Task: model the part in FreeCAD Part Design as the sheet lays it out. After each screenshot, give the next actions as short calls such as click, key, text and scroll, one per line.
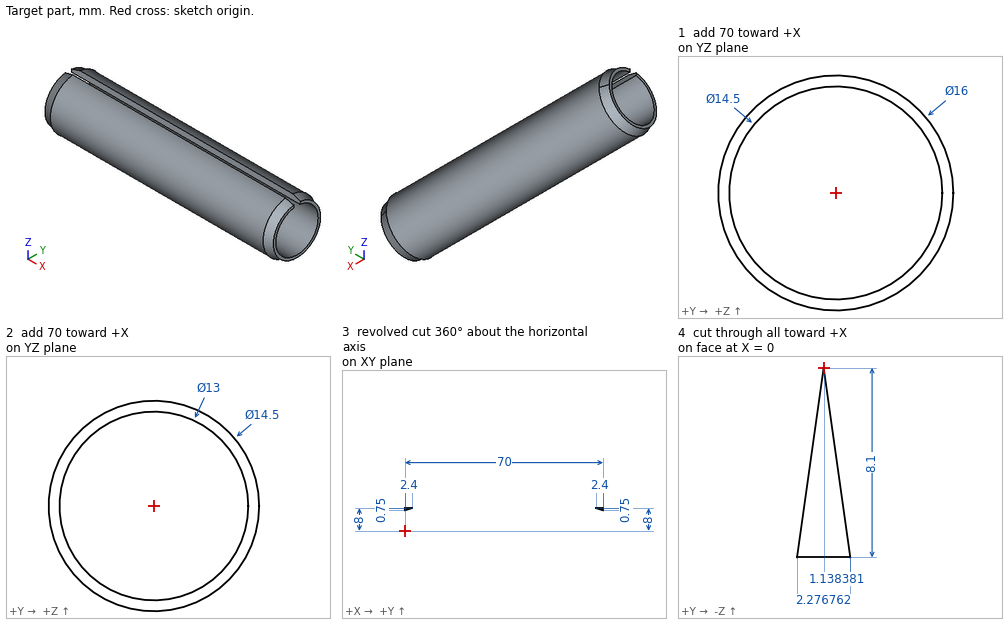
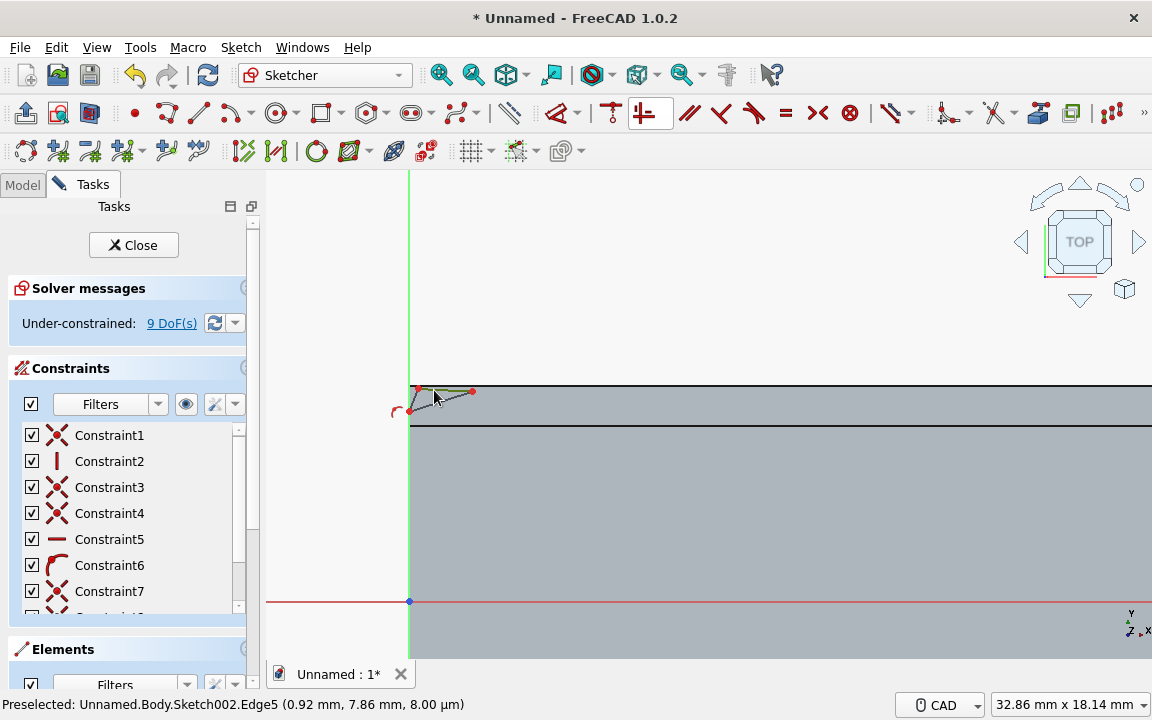
key(h)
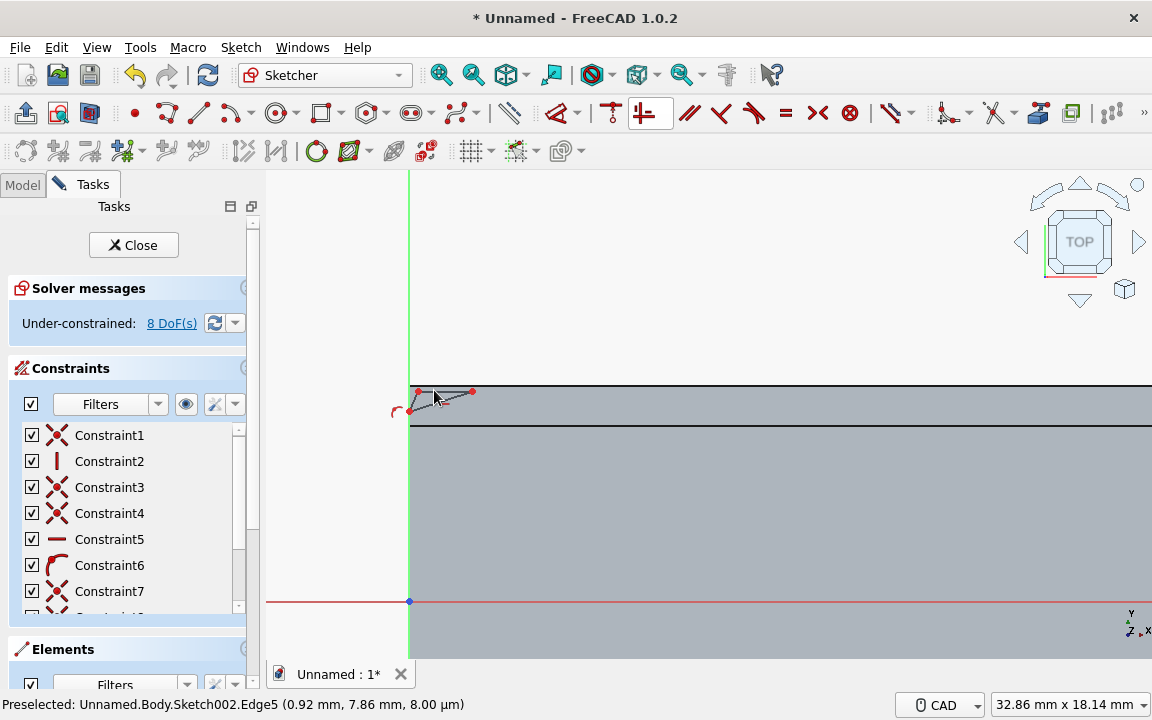
scroll(413, 404, up, 4)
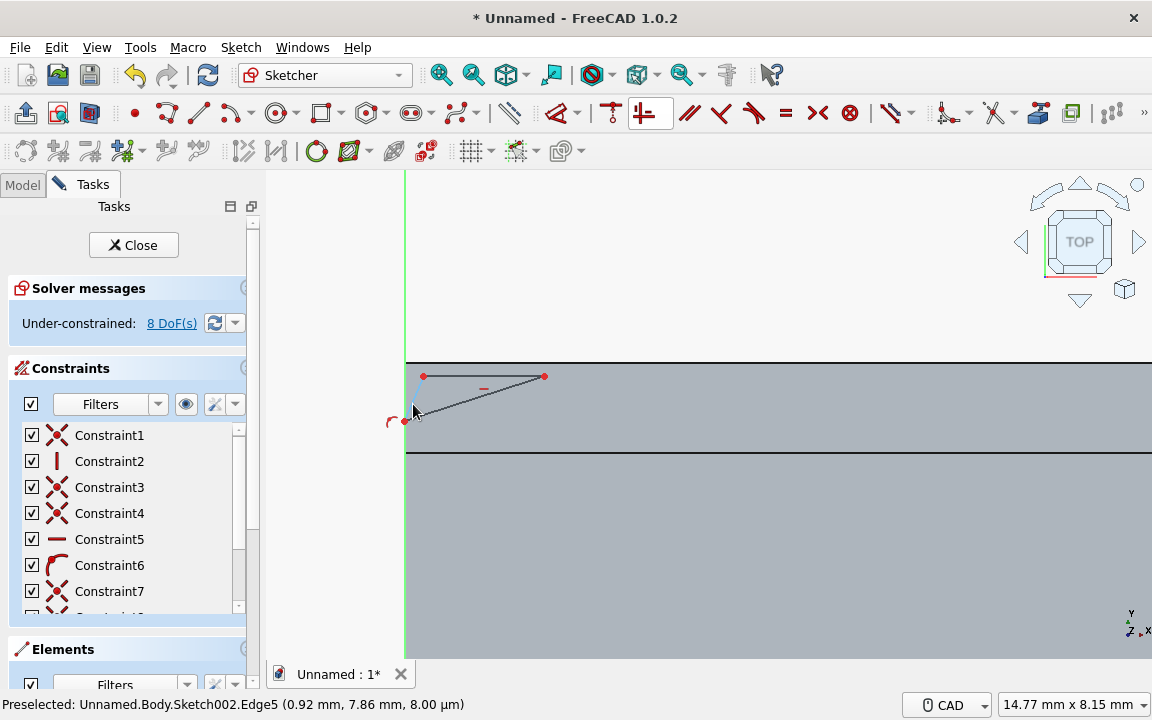
click(412, 403)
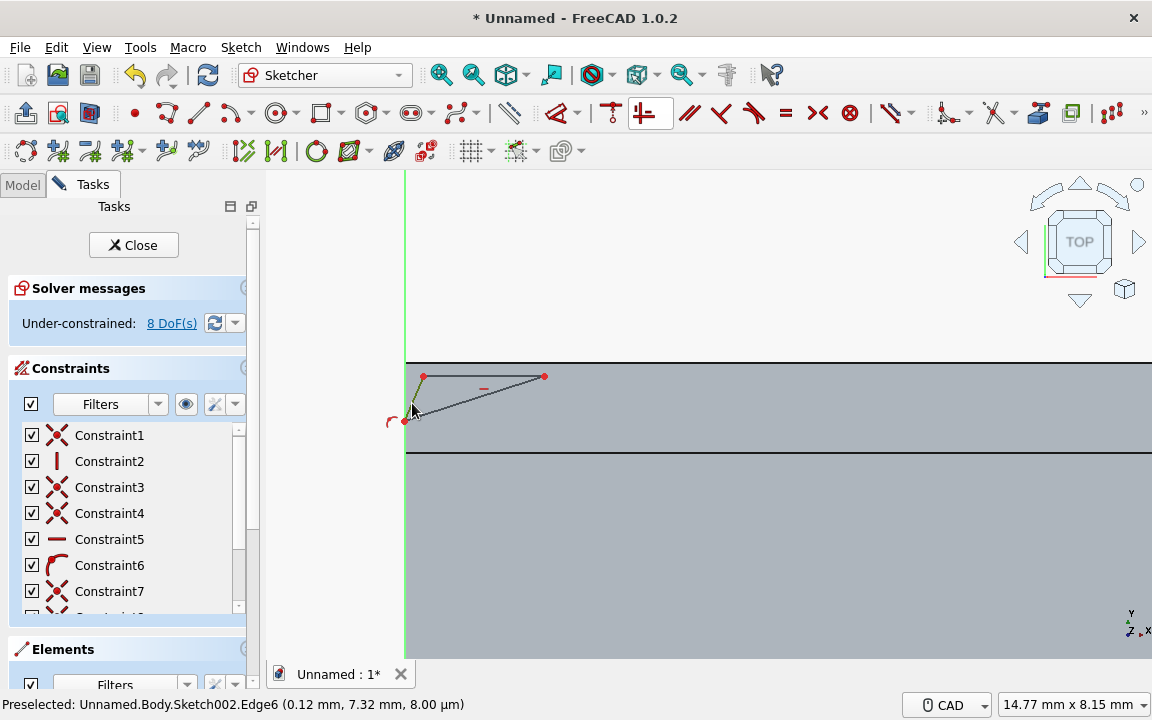
key(v)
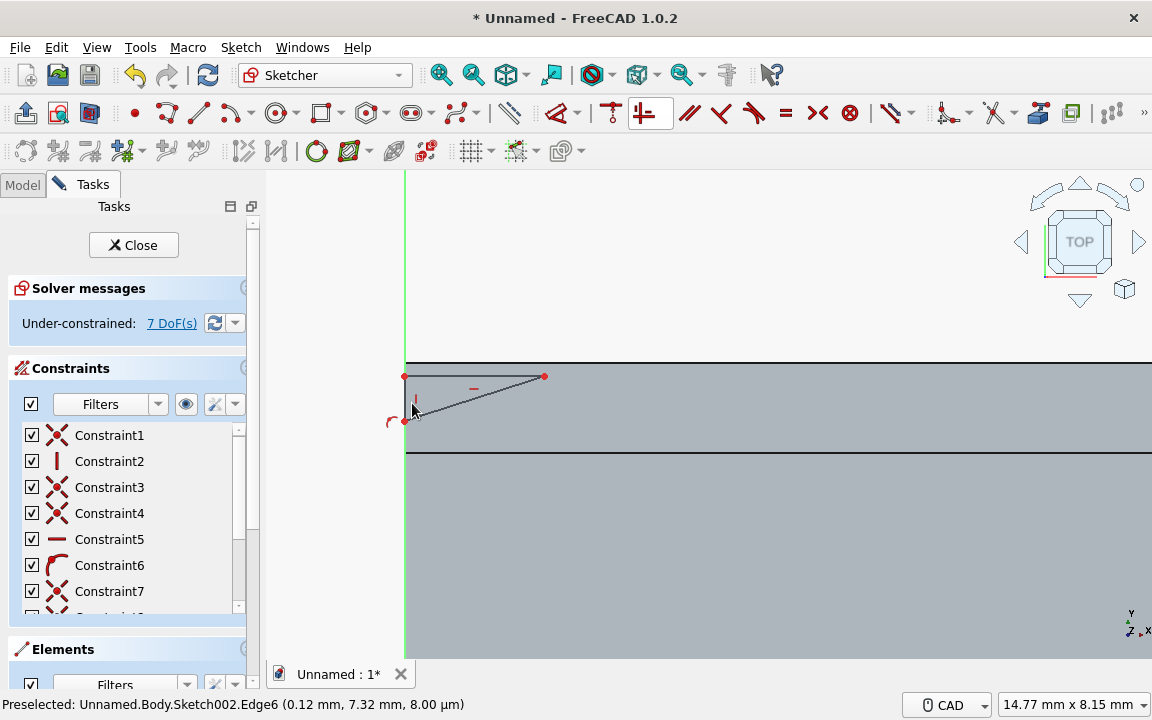
click(556, 114)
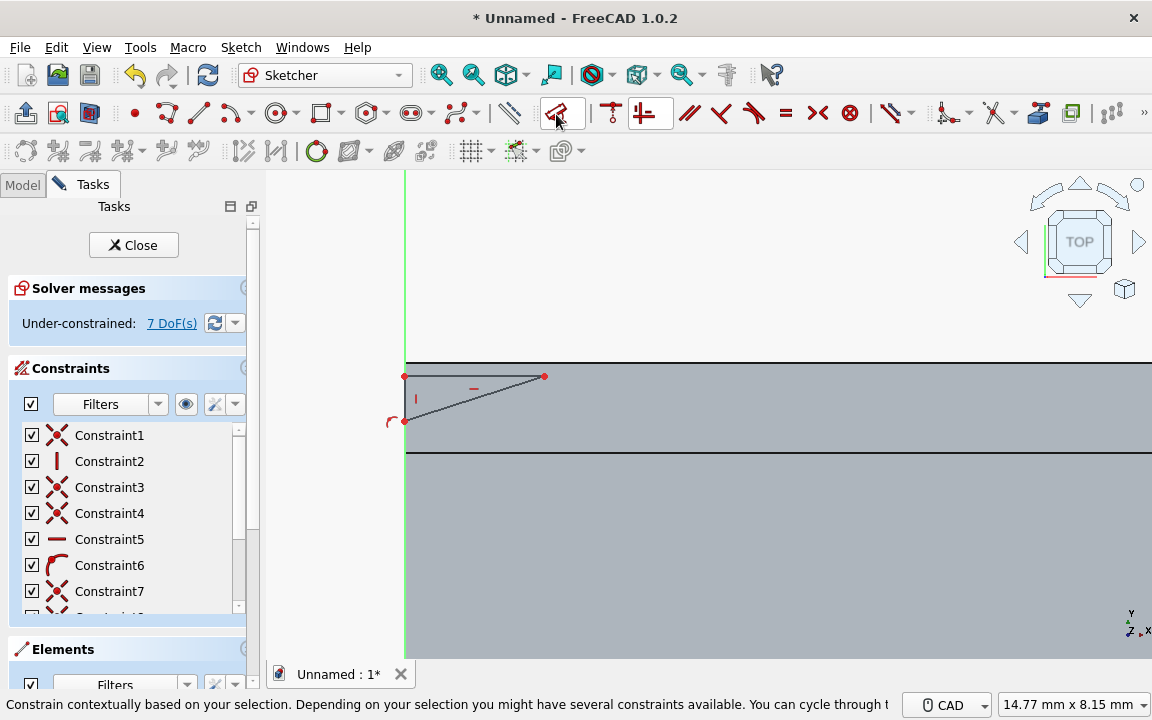
scroll(408, 391, down, 11)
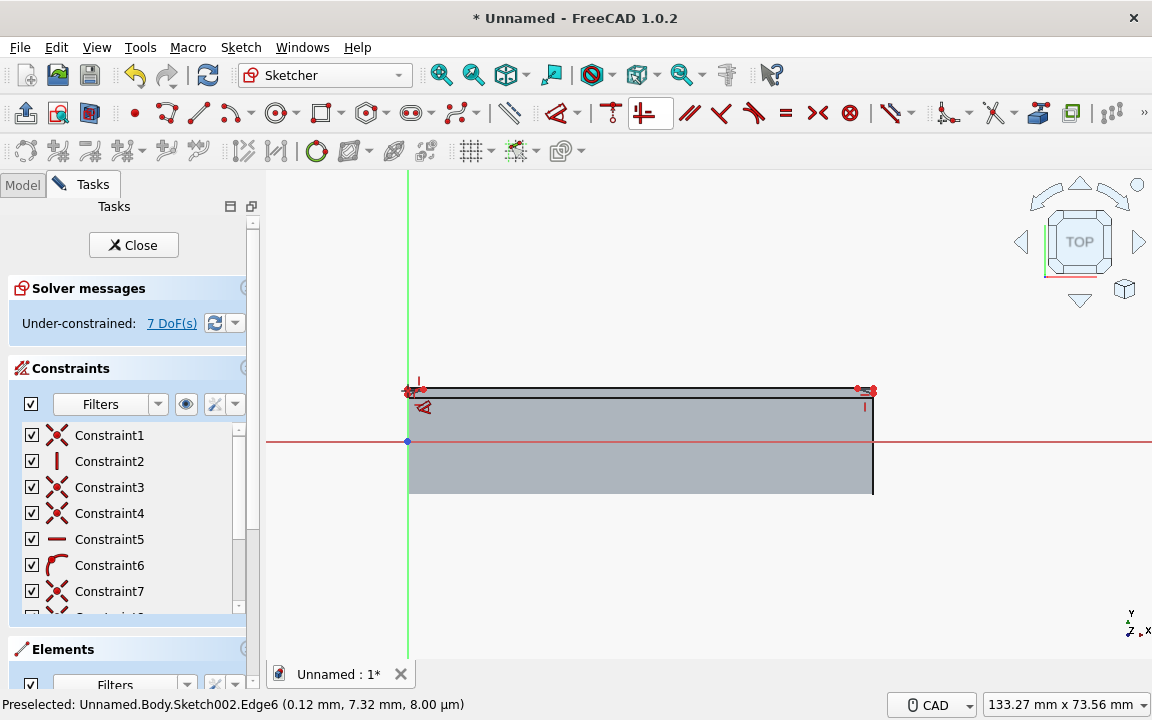
click(857, 389)
click(374, 415)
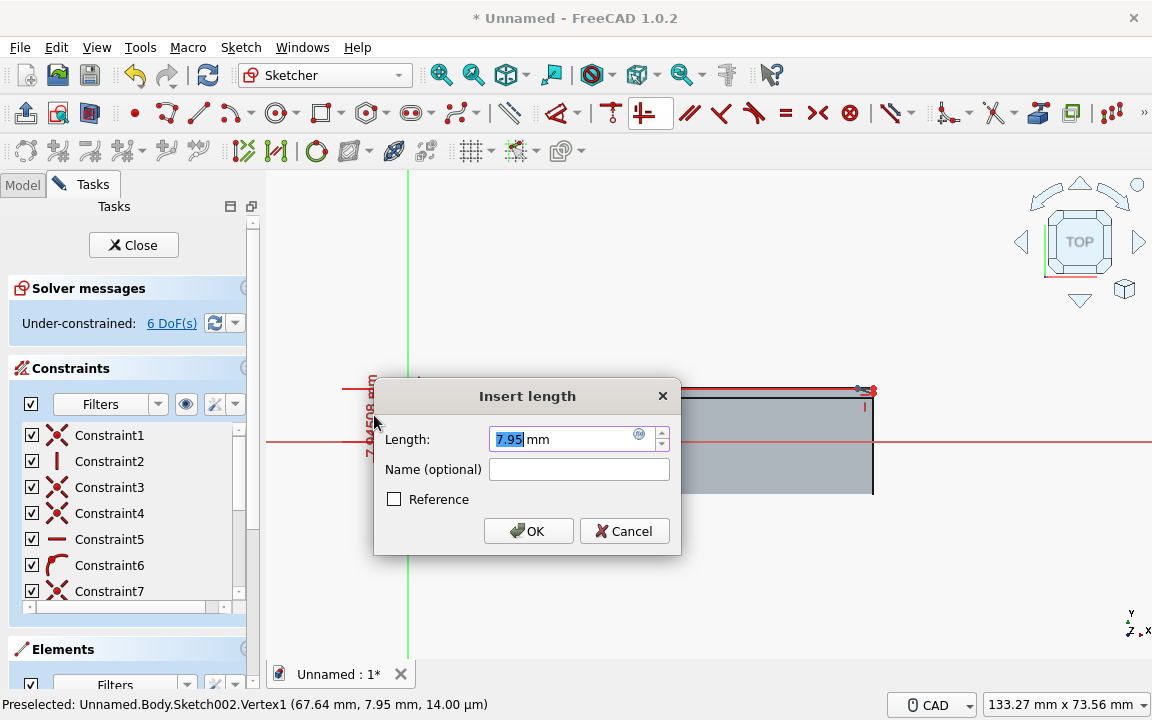
text(8)
key(Return)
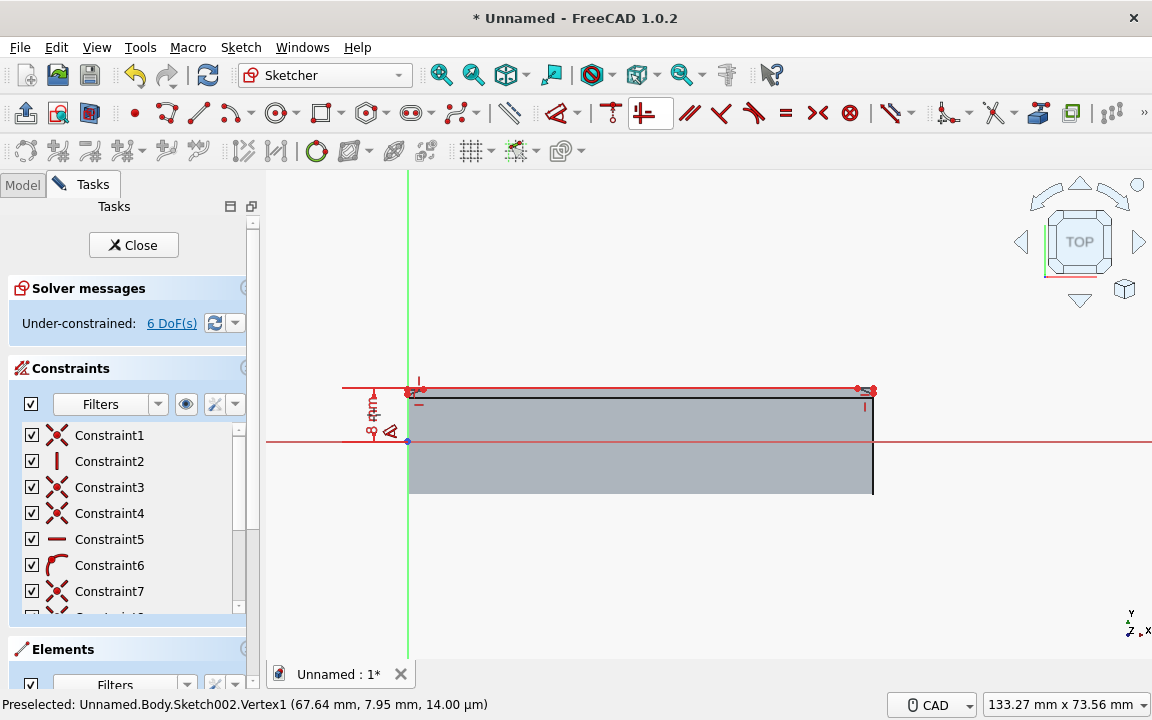
click(423, 390)
click(457, 416)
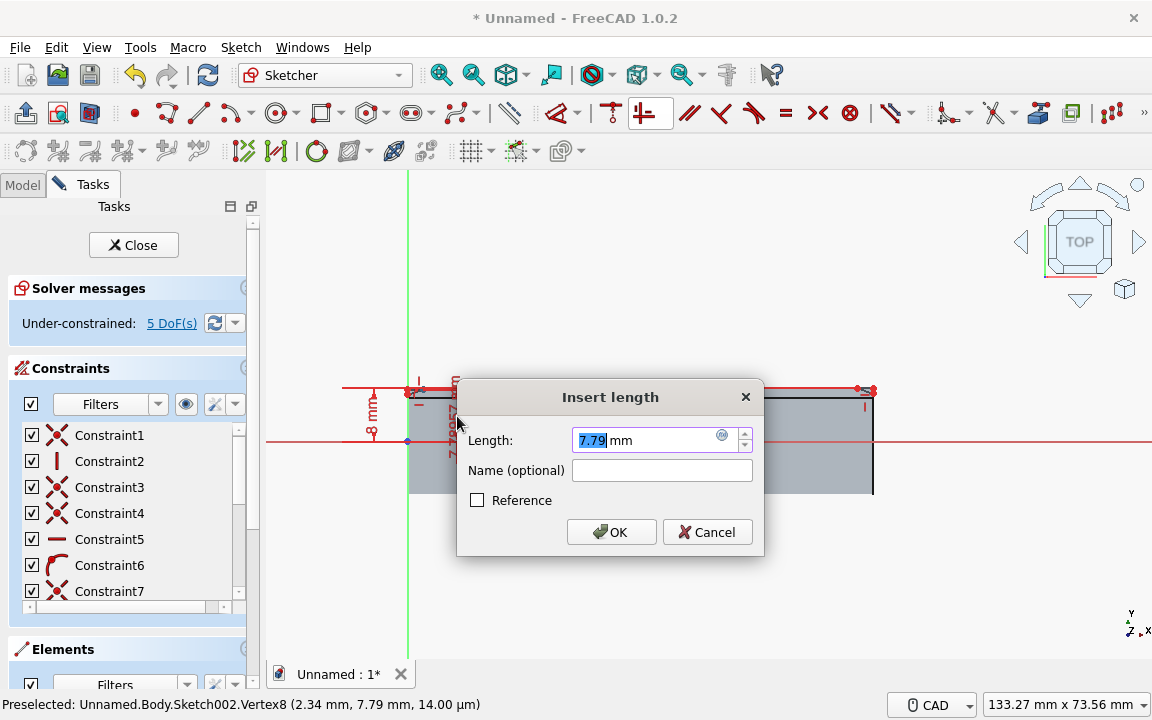
text(8)
key(Return)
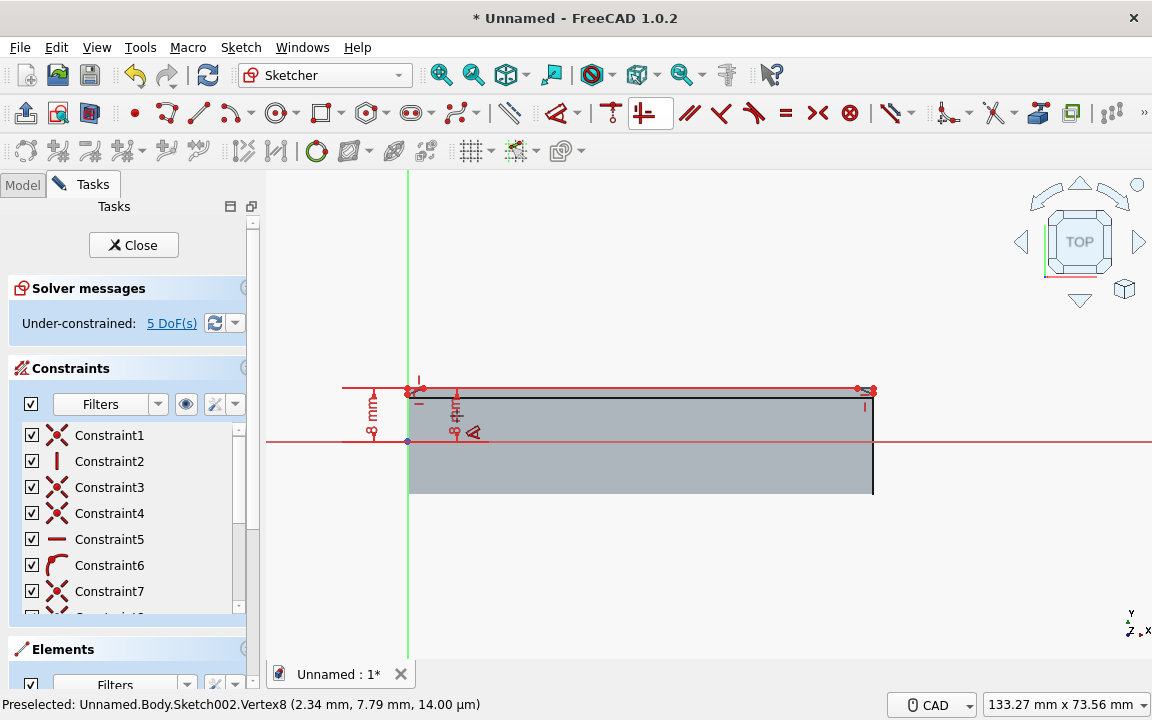
scroll(869, 388, up, 7)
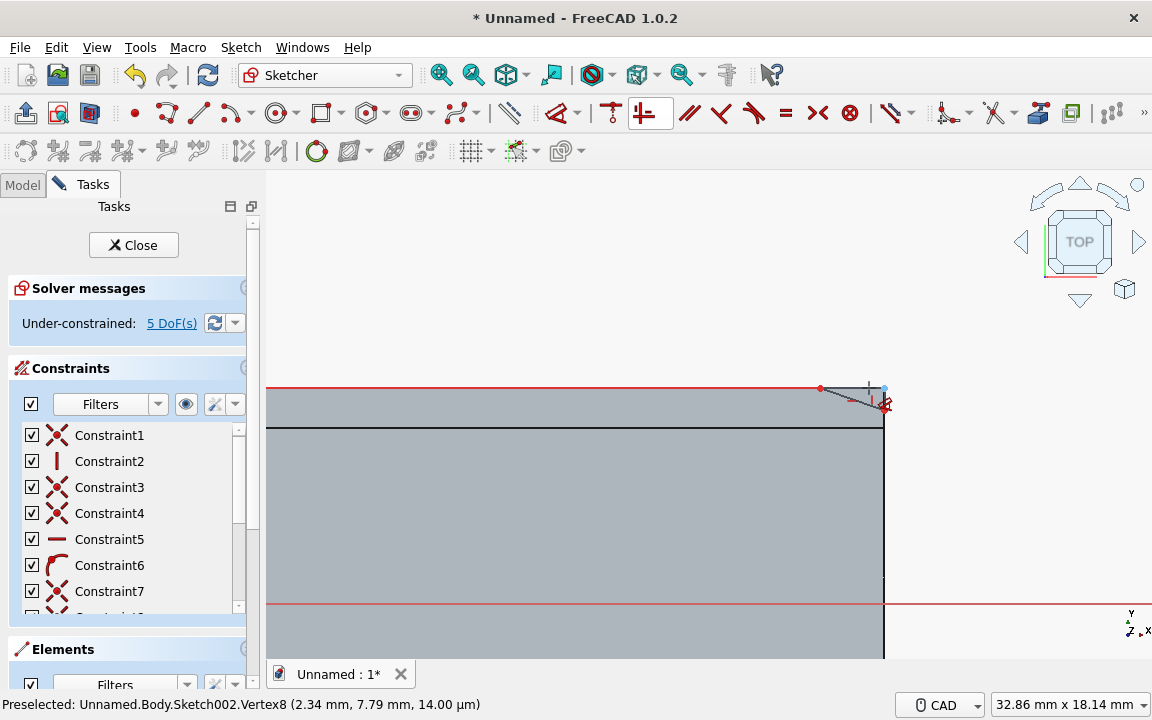
click(865, 388)
click(852, 354)